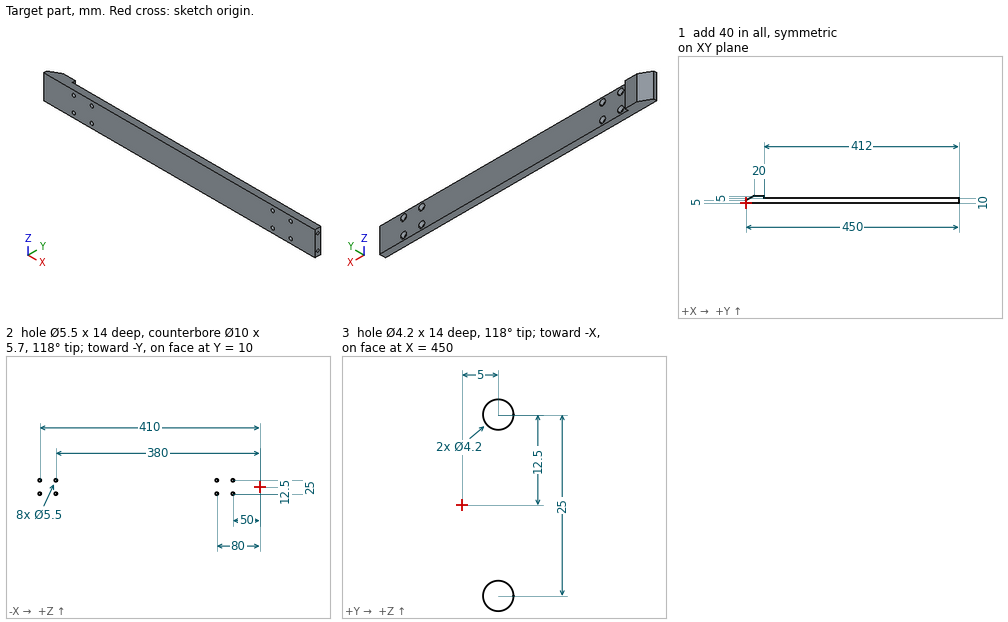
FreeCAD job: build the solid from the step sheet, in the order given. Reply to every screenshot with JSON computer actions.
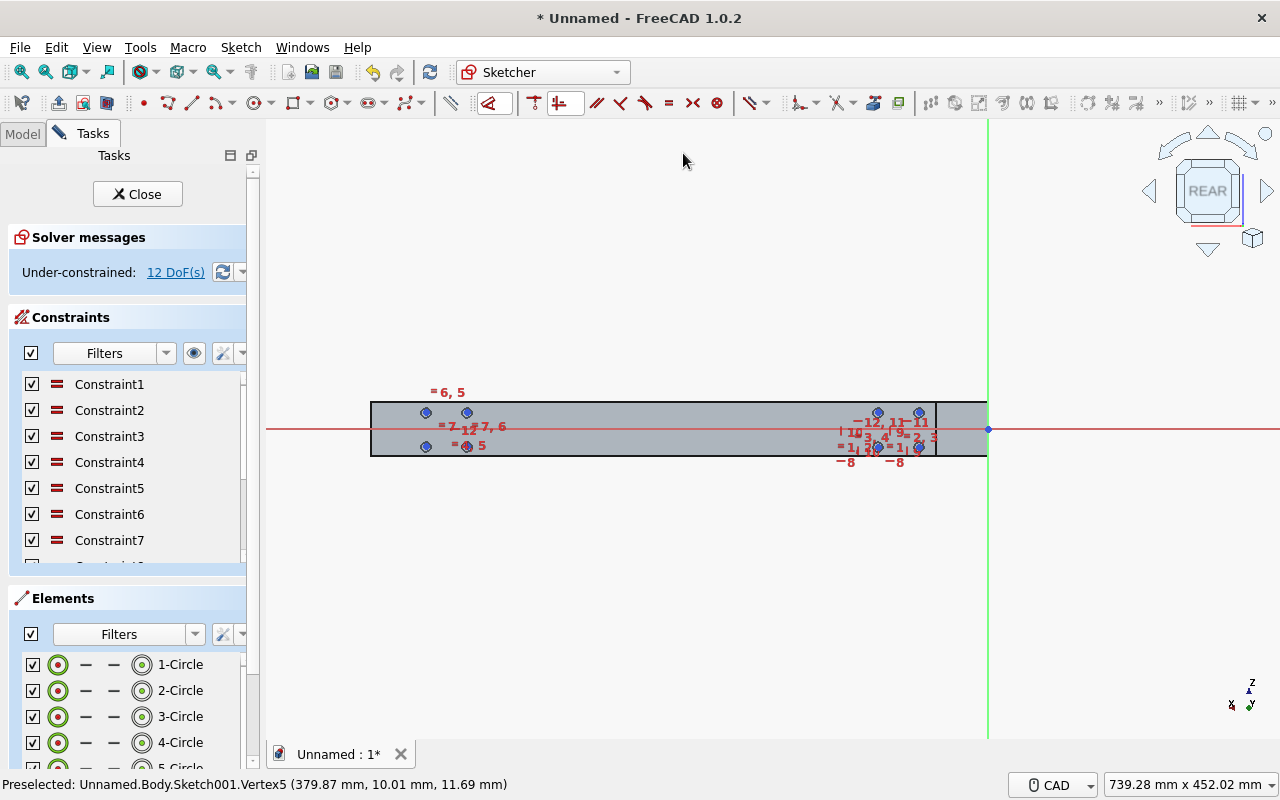
{"action": "left_click", "coordinate": [467, 413]}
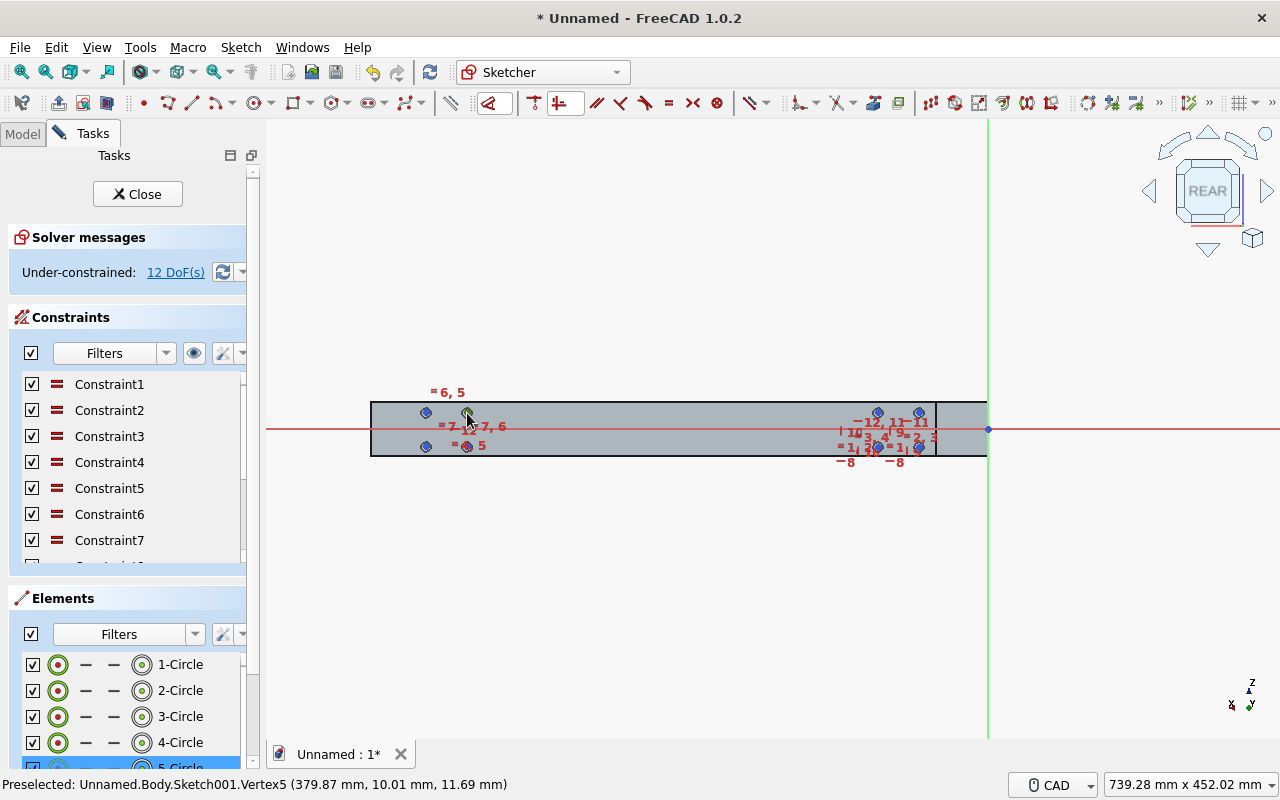
{"action": "left_click", "coordinate": [426, 413]}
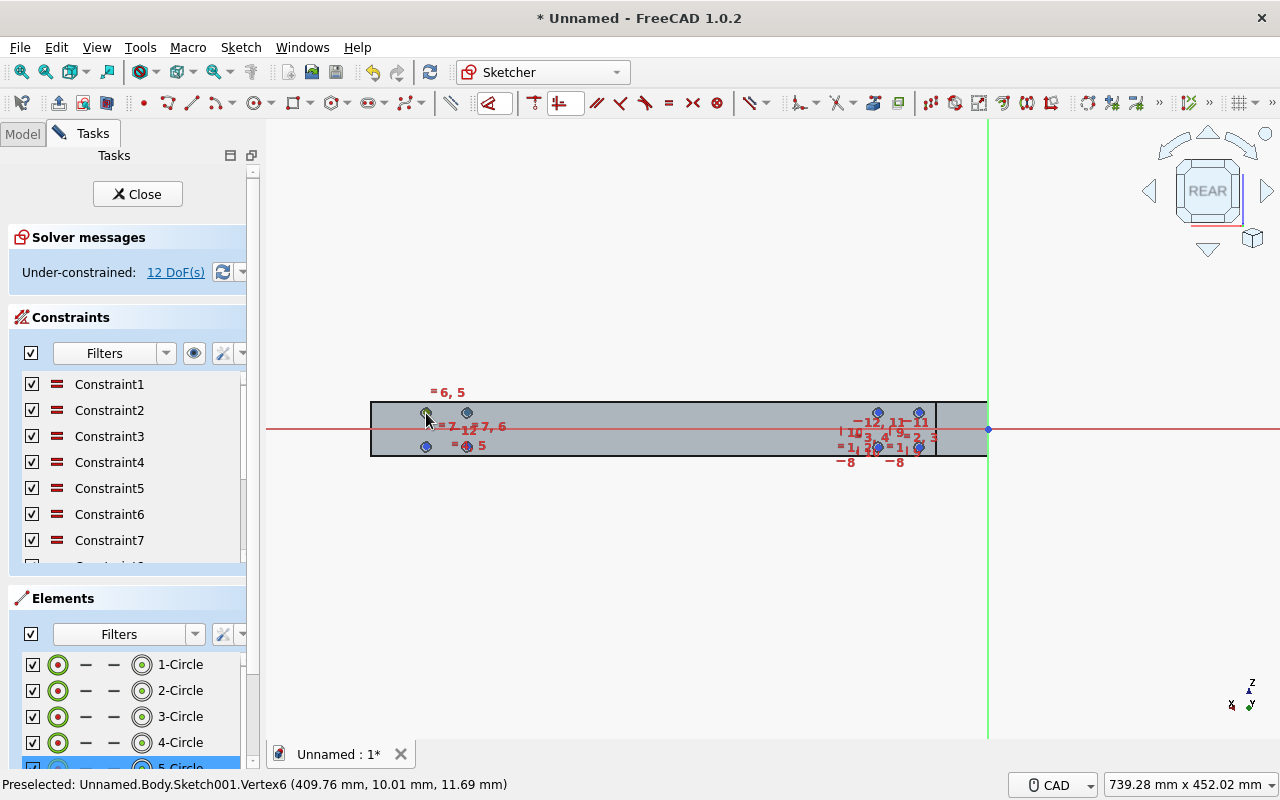
{"action": "left_click", "coordinate": [578, 104]}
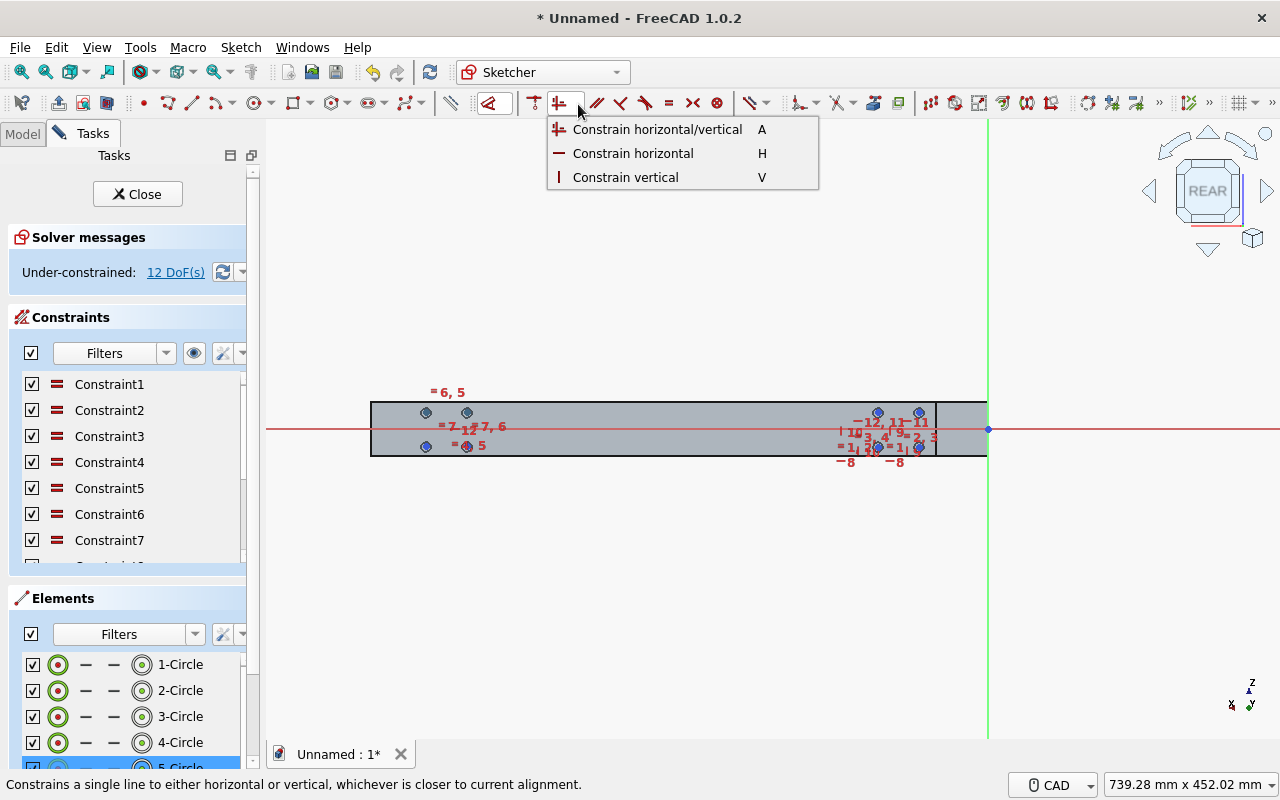
{"action": "left_click", "coordinate": [683, 153]}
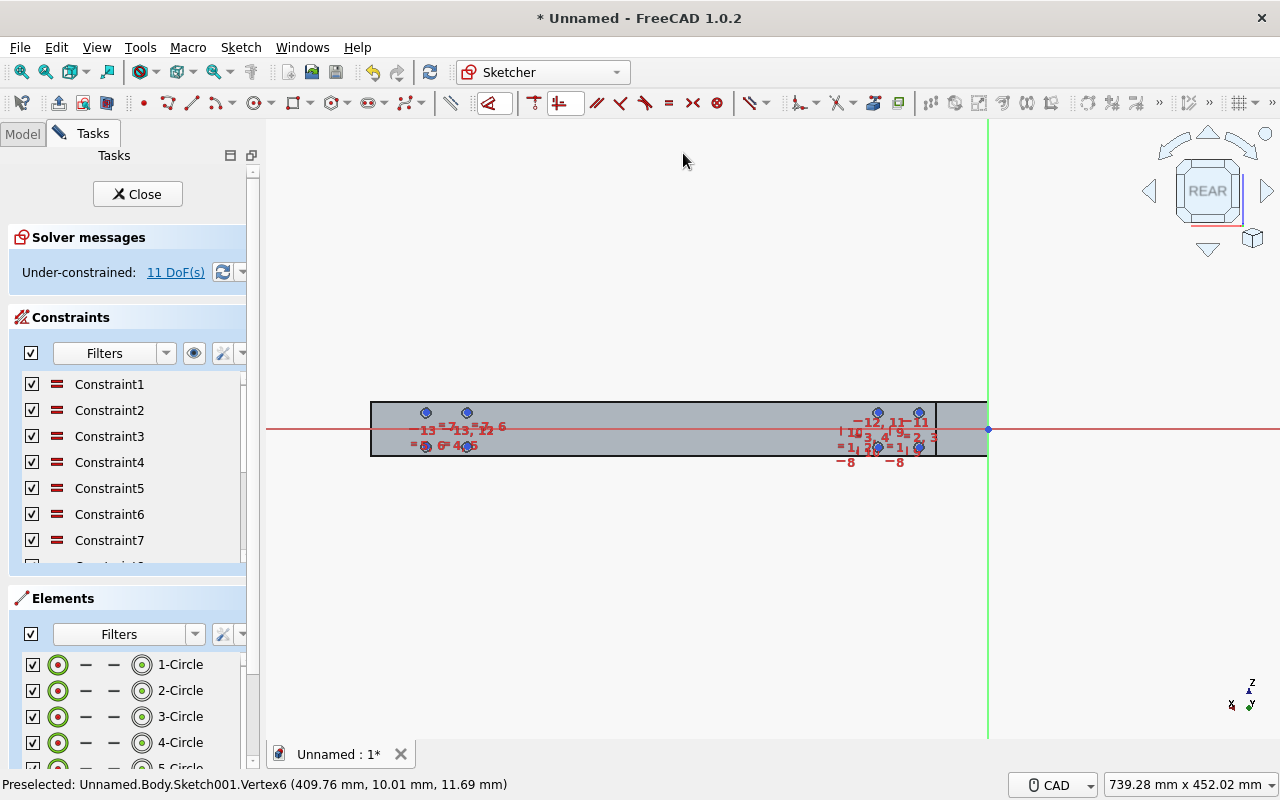
{"action": "left_click", "coordinate": [467, 413]}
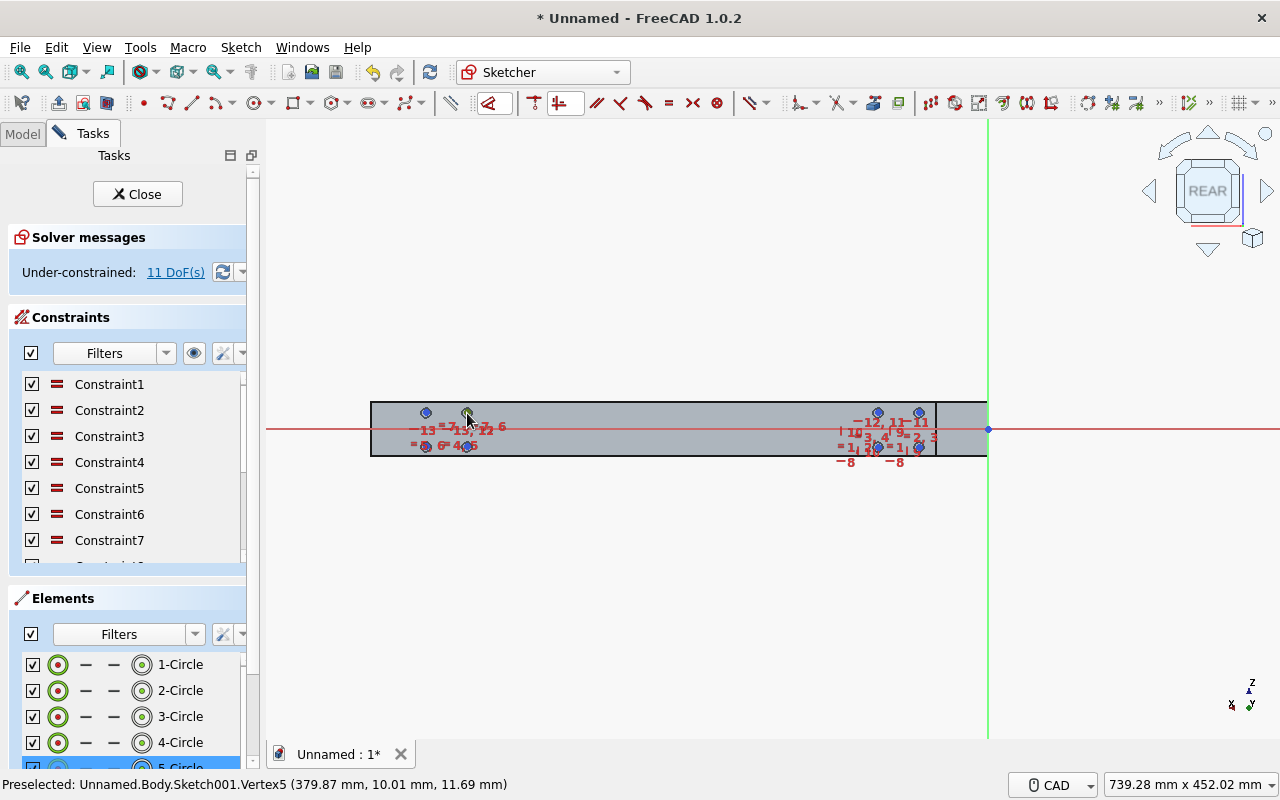
{"action": "left_click", "coordinate": [467, 447]}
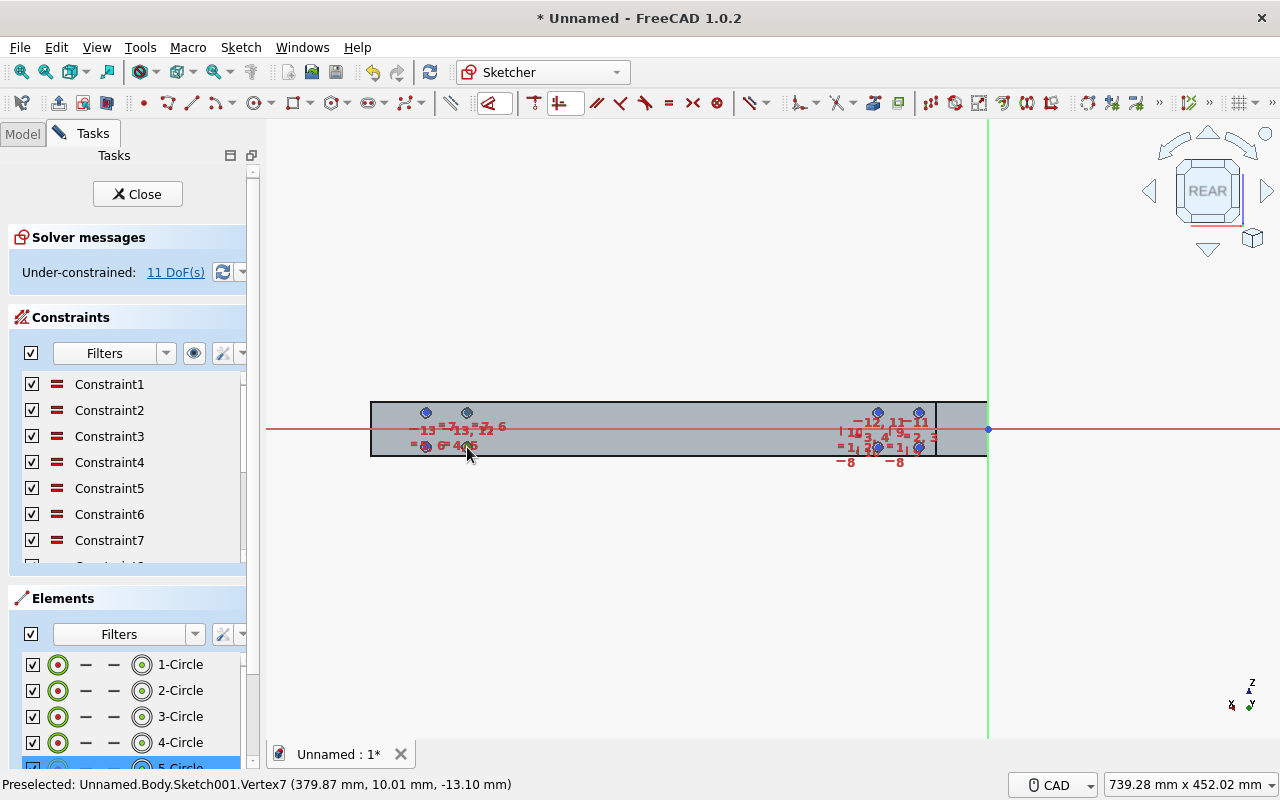
{"action": "left_click", "coordinate": [578, 104]}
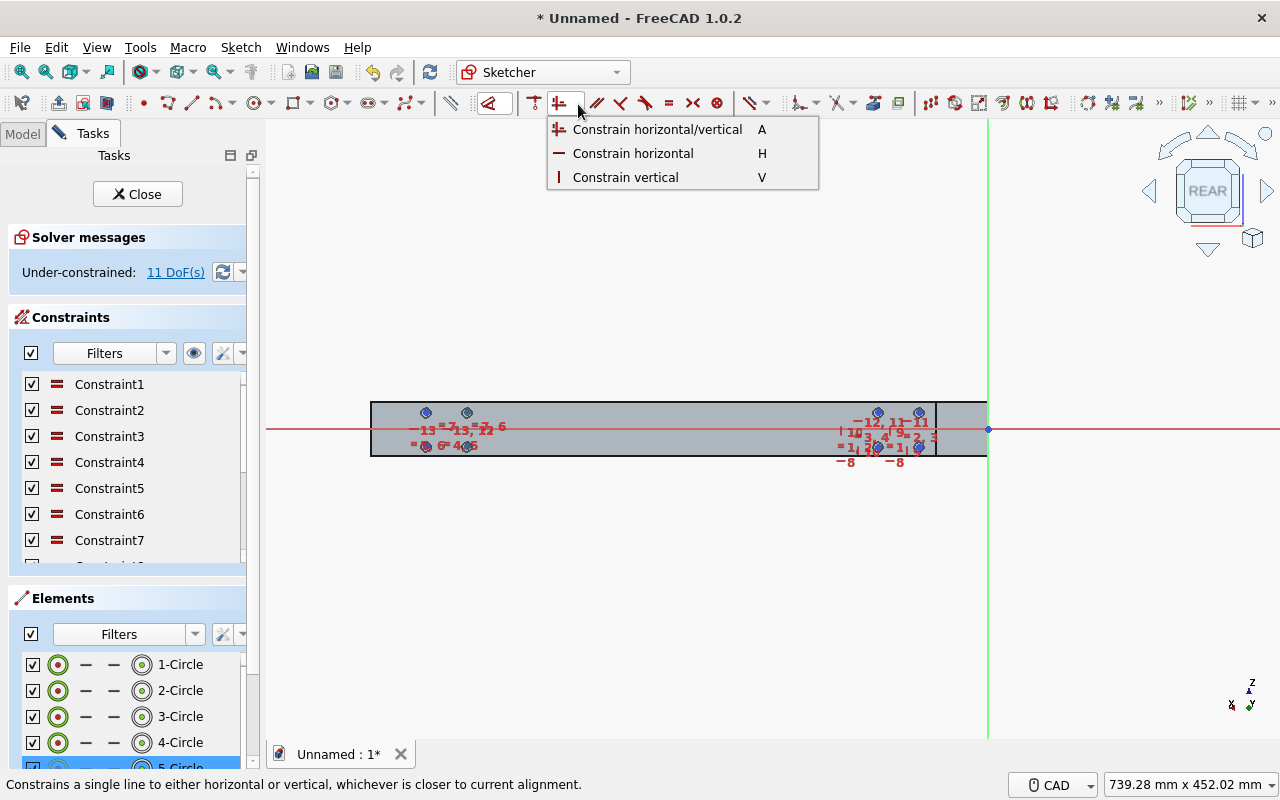
{"action": "left_click", "coordinate": [683, 177]}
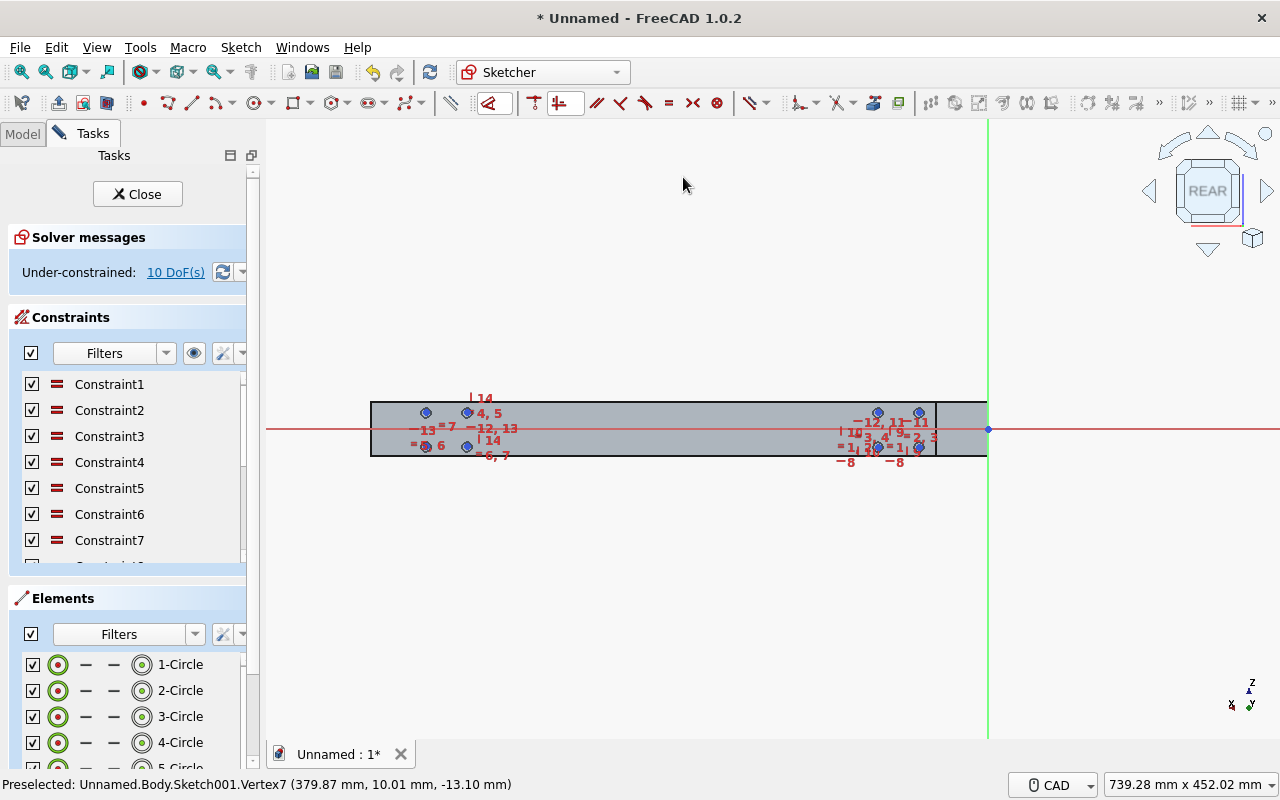
{"action": "left_click", "coordinate": [878, 447]}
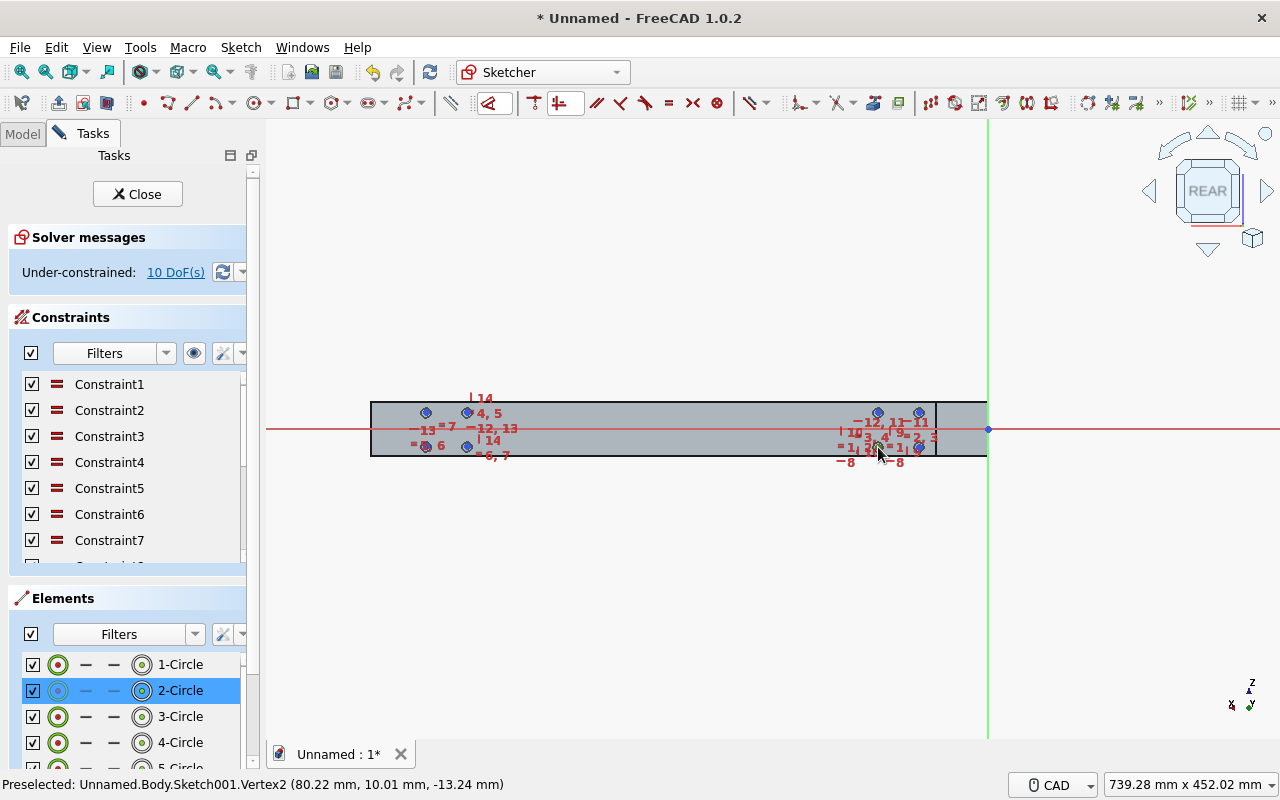
{"action": "left_click", "coordinate": [467, 447]}